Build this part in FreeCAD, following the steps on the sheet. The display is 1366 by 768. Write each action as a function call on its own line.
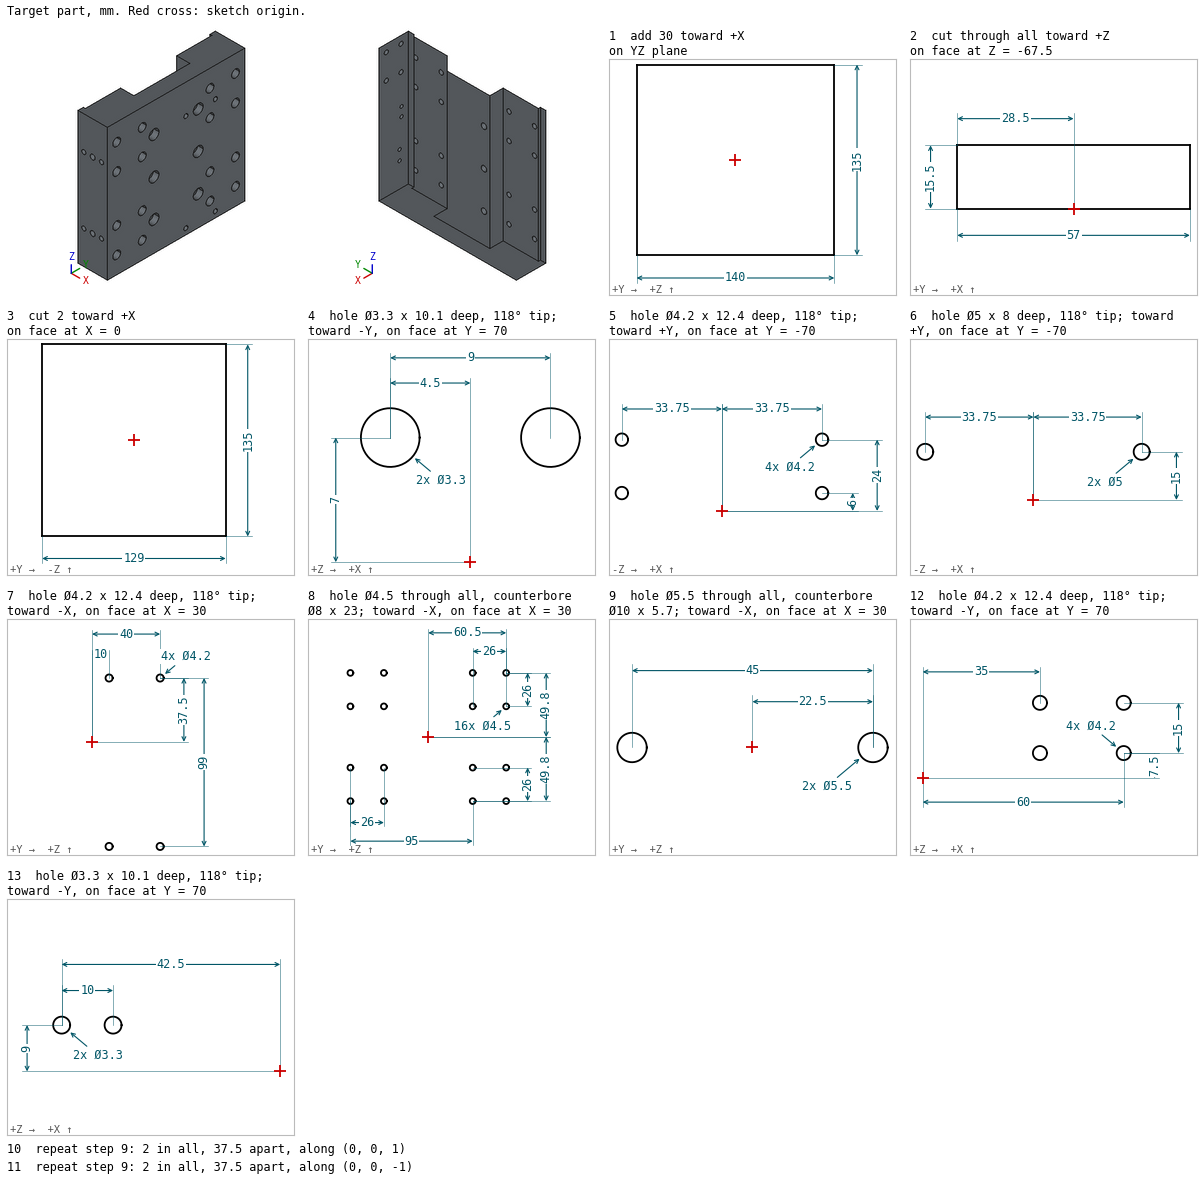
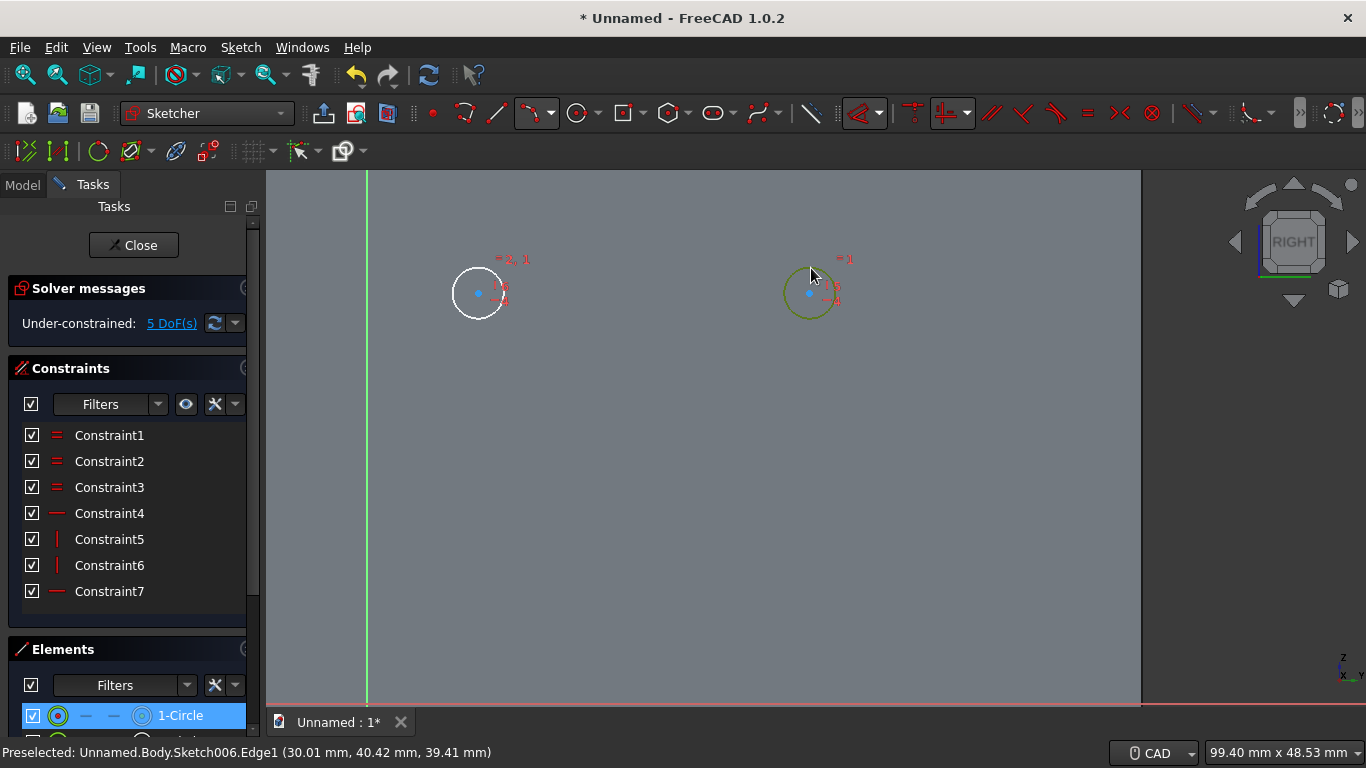
key(k)
key(o)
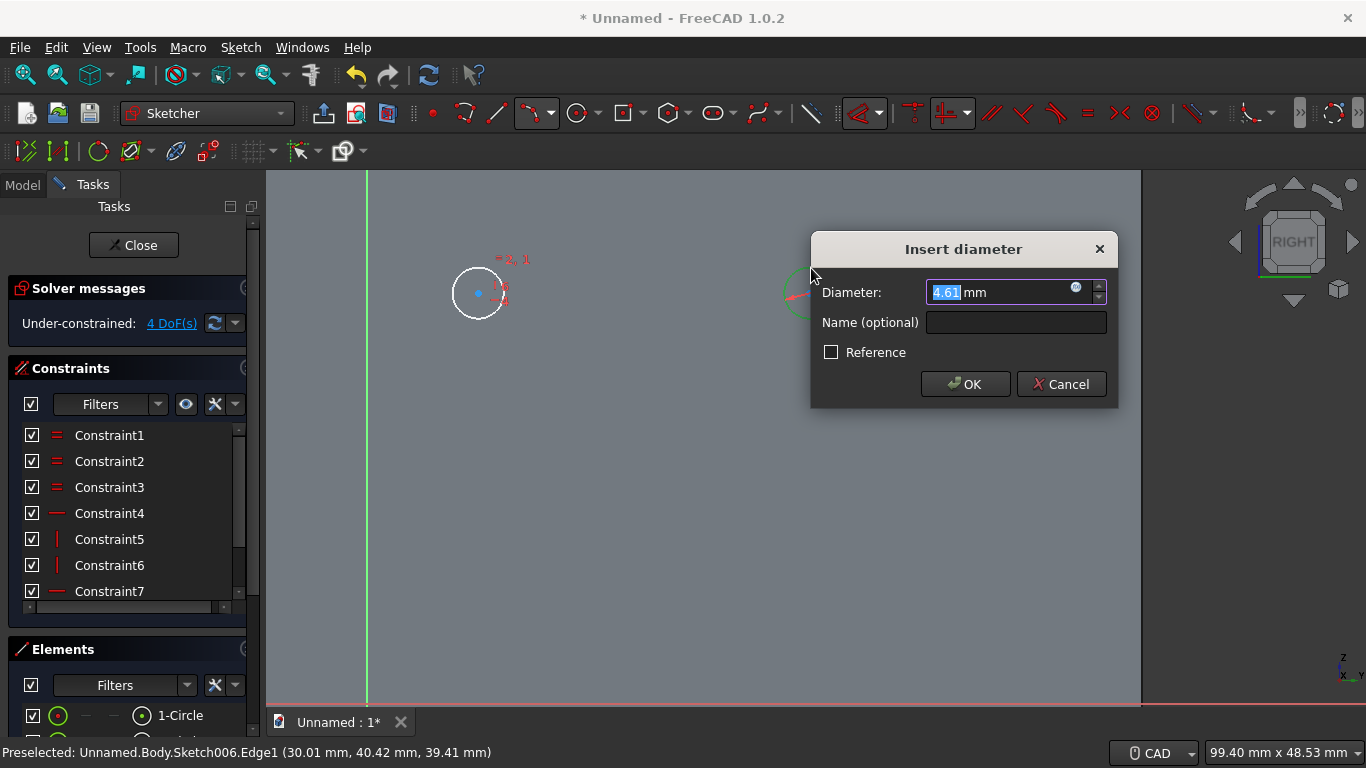
text(4.2)
key(Return)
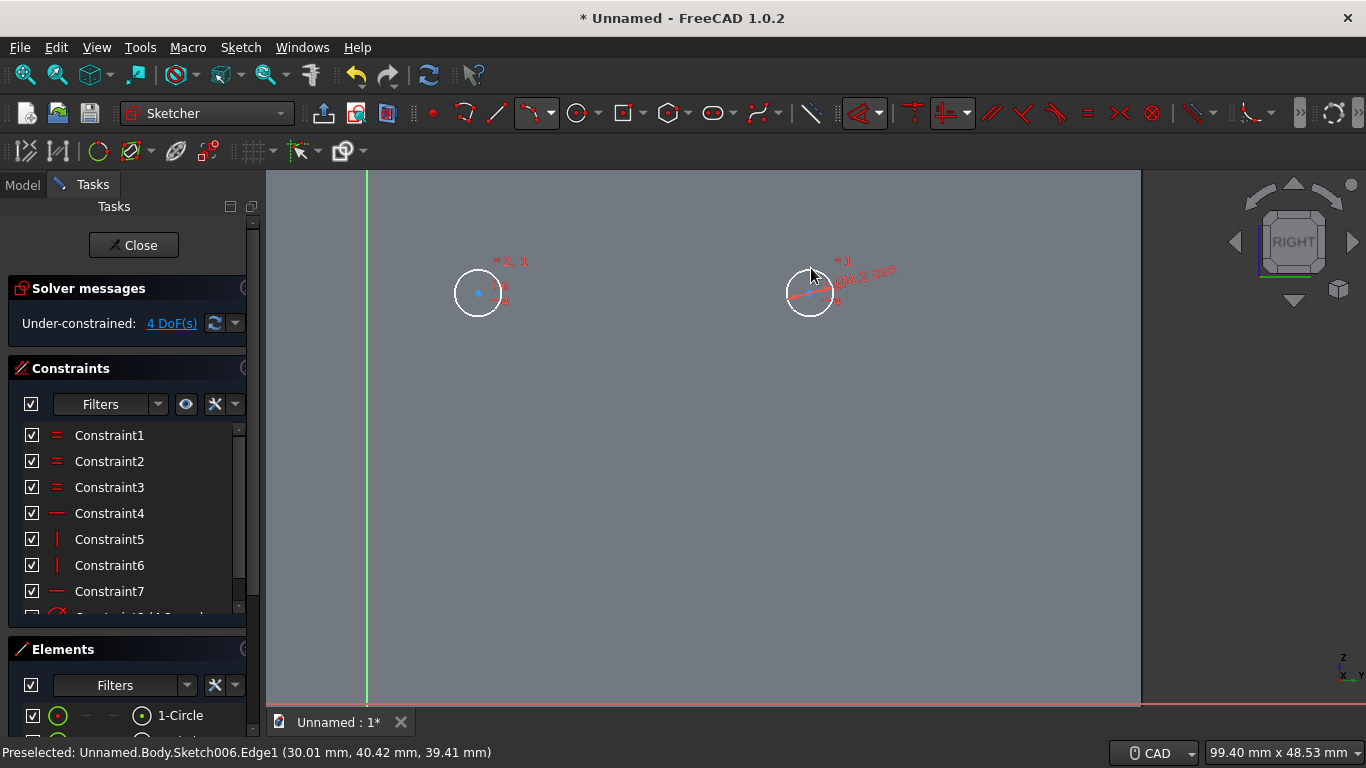
scroll(811, 267, down, 6)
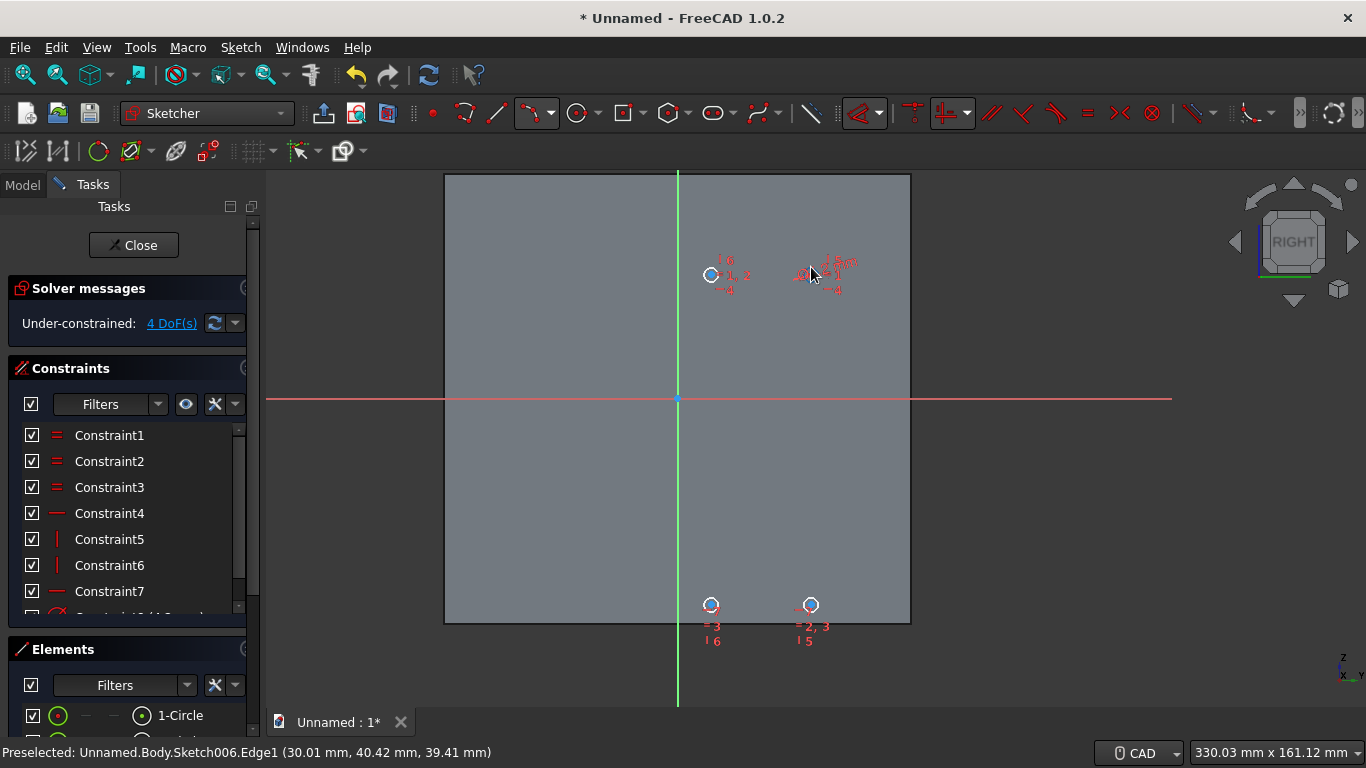
click(811, 275)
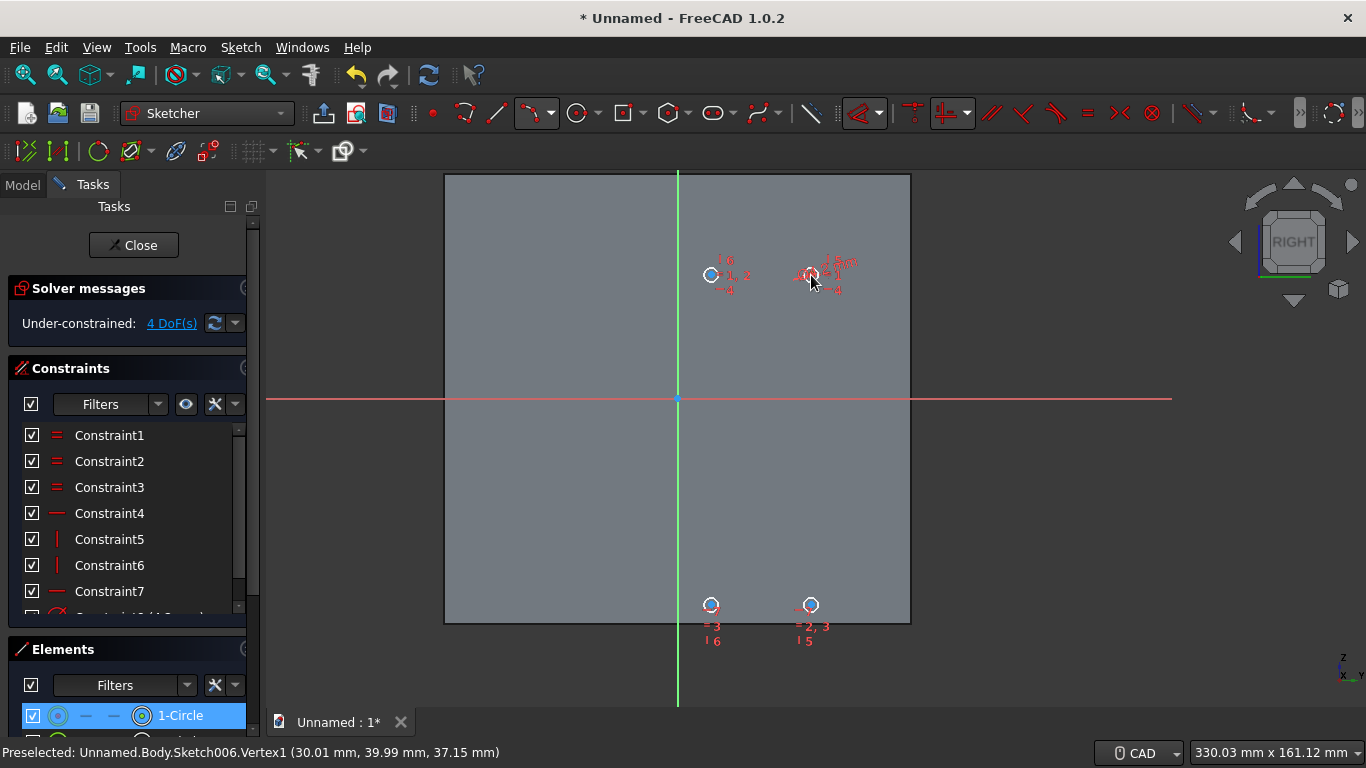
click(882, 114)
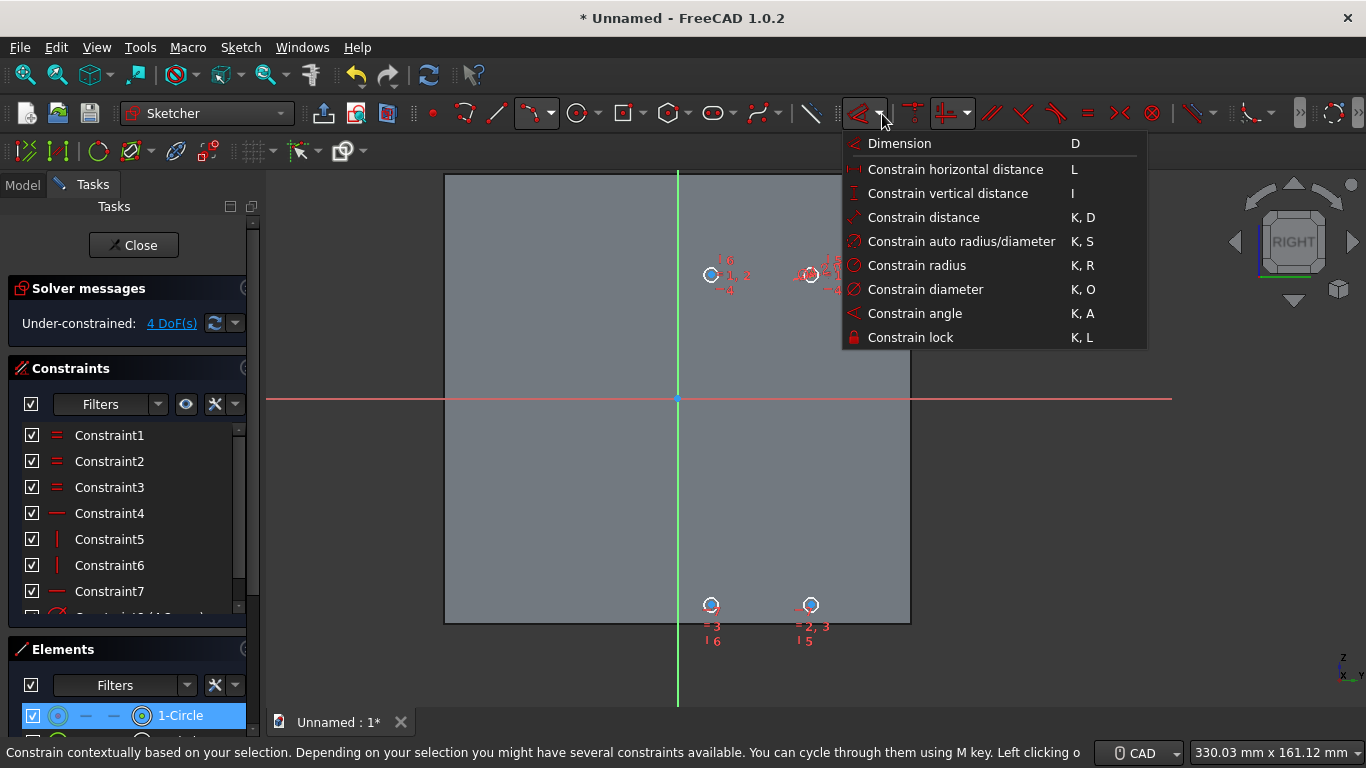
click(995, 169)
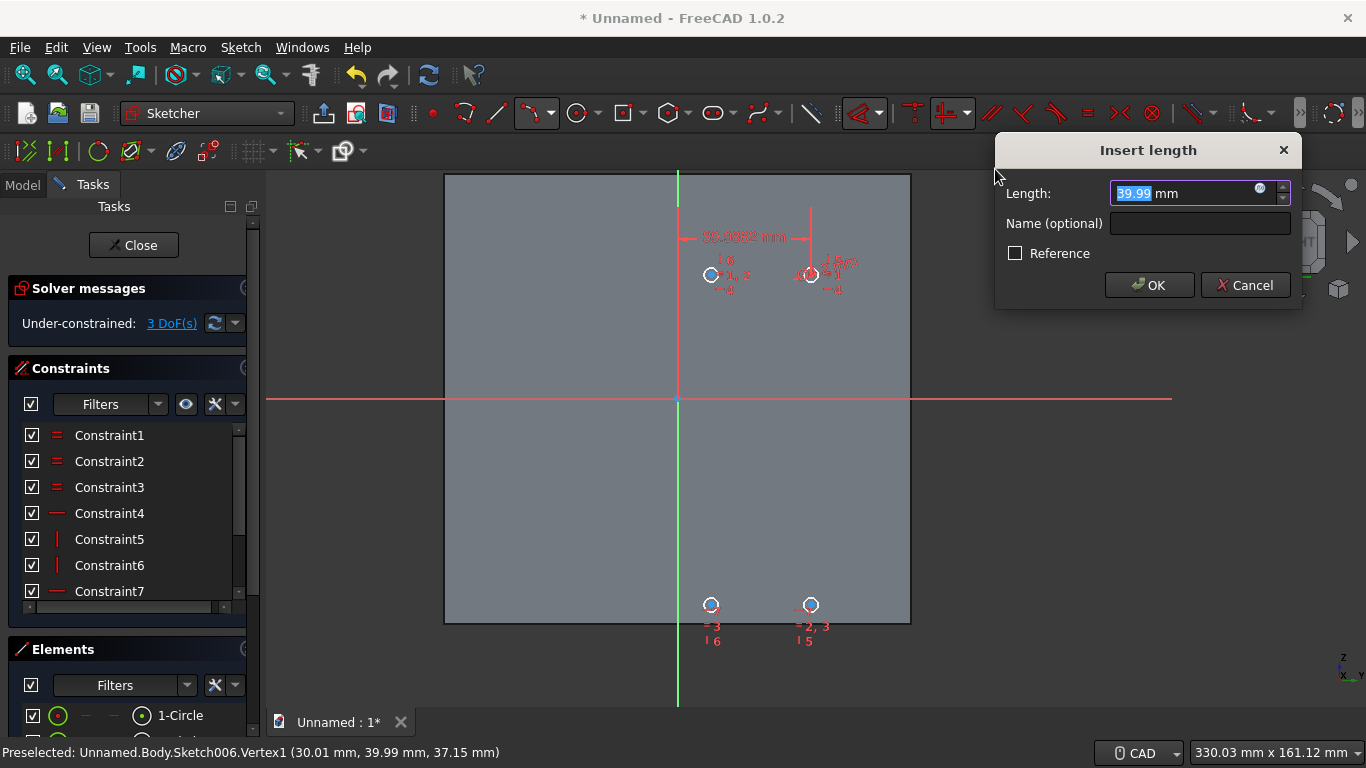
text(40)
key(Return)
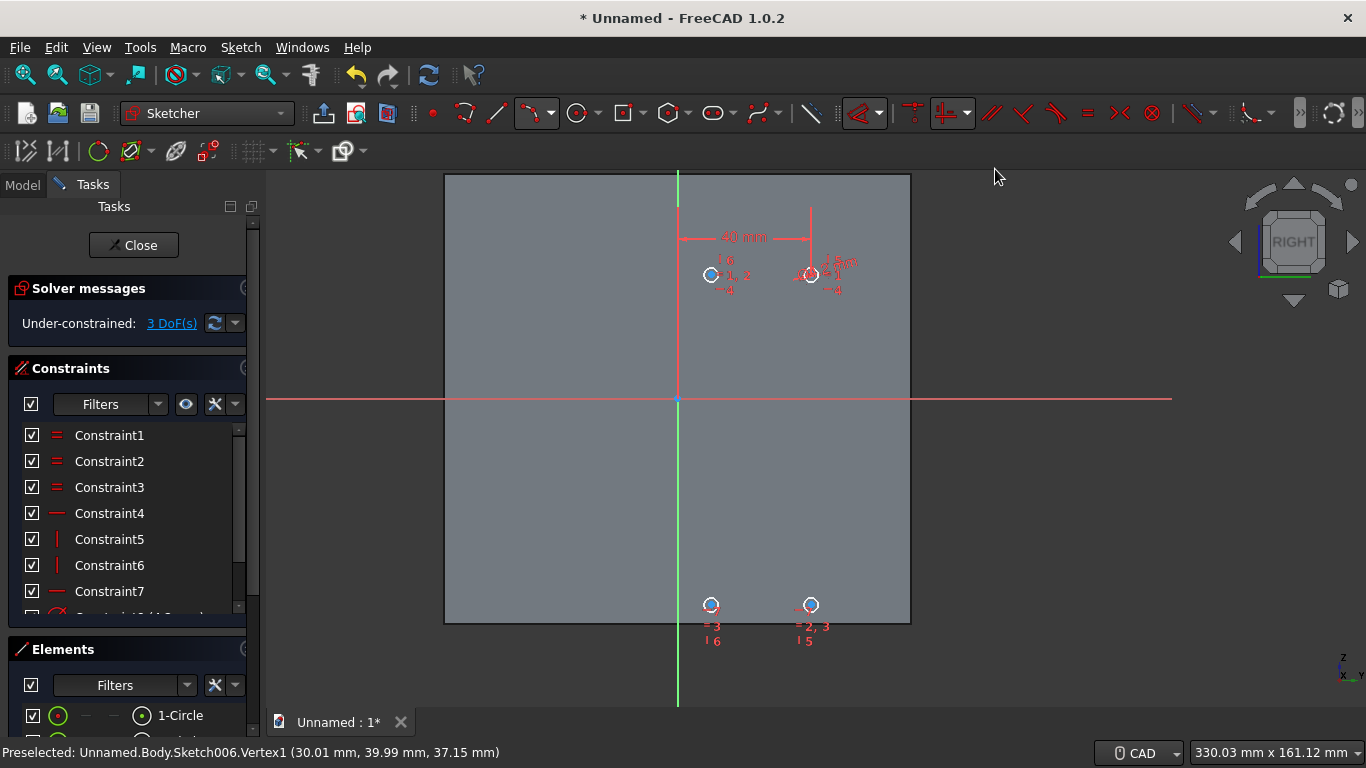
click(711, 275)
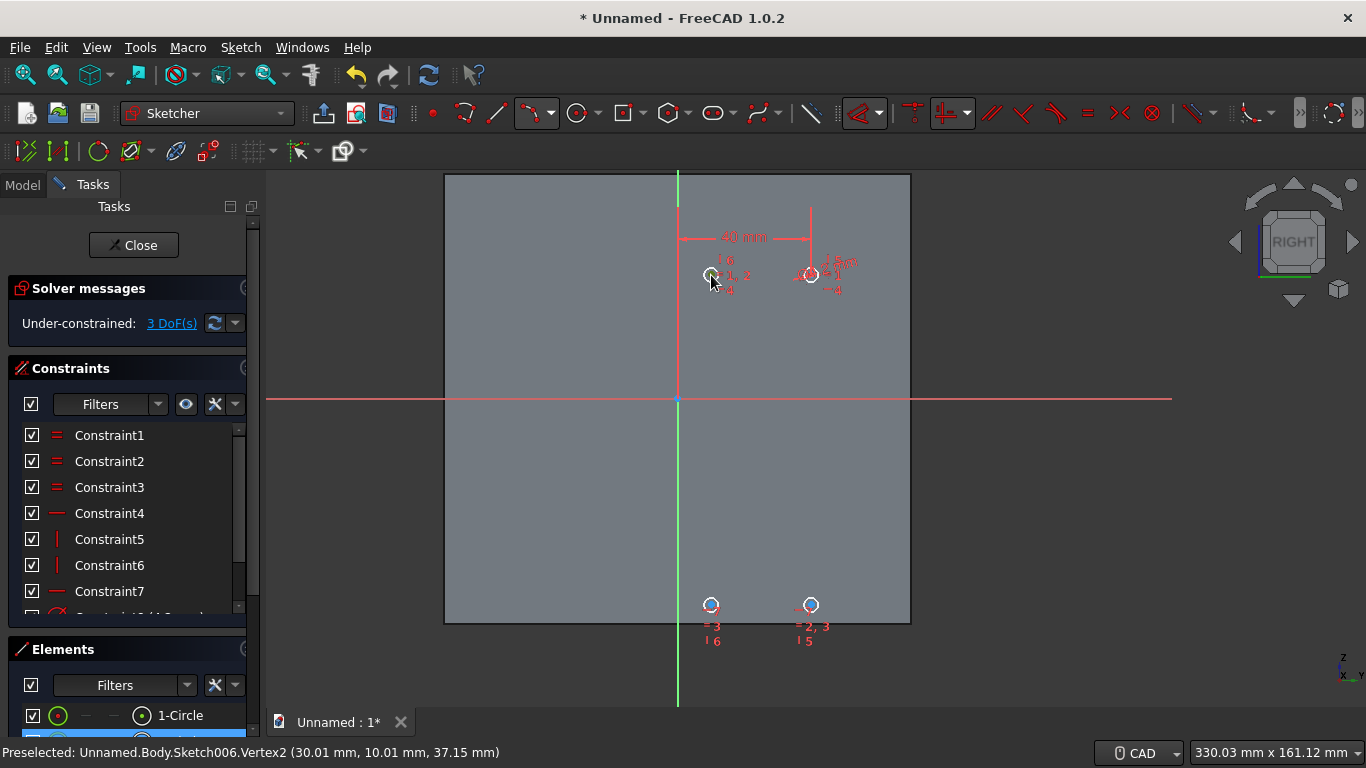
click(882, 114)